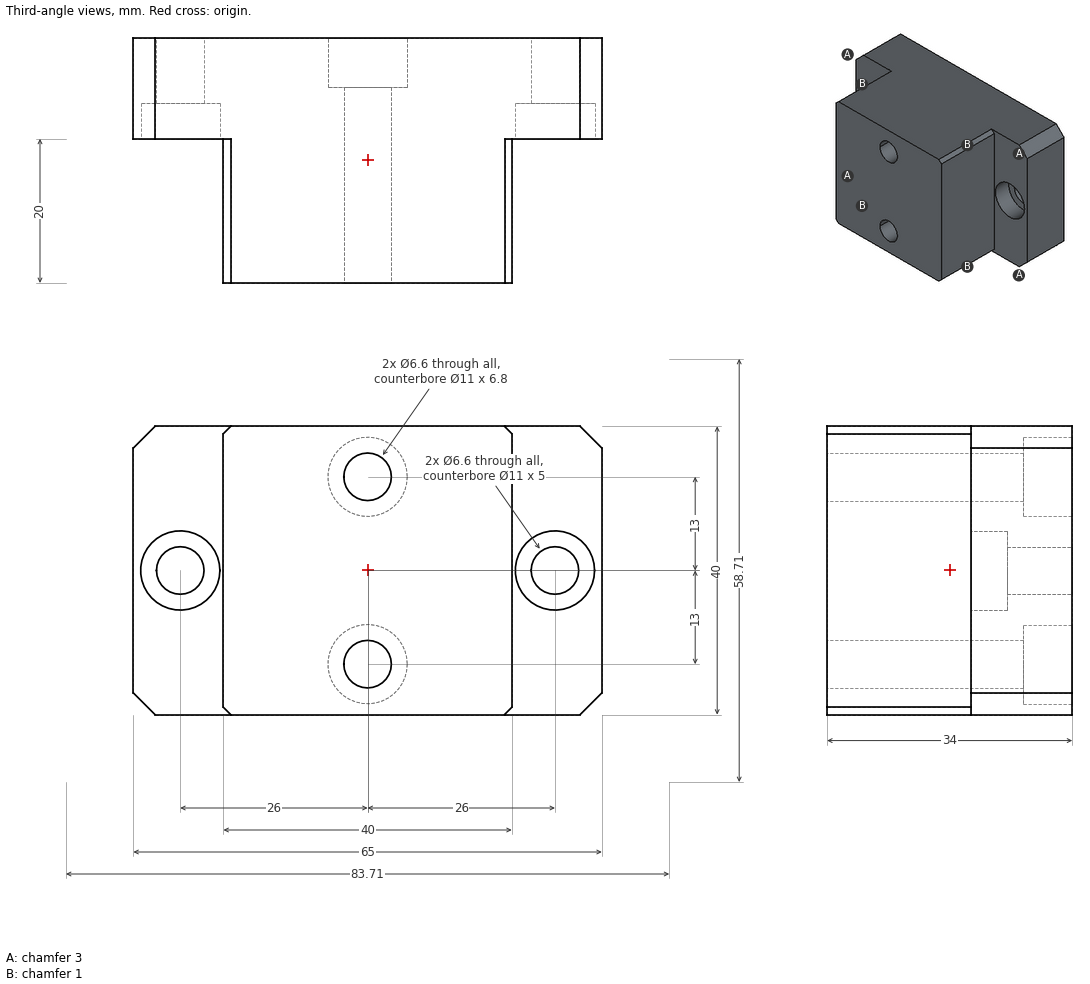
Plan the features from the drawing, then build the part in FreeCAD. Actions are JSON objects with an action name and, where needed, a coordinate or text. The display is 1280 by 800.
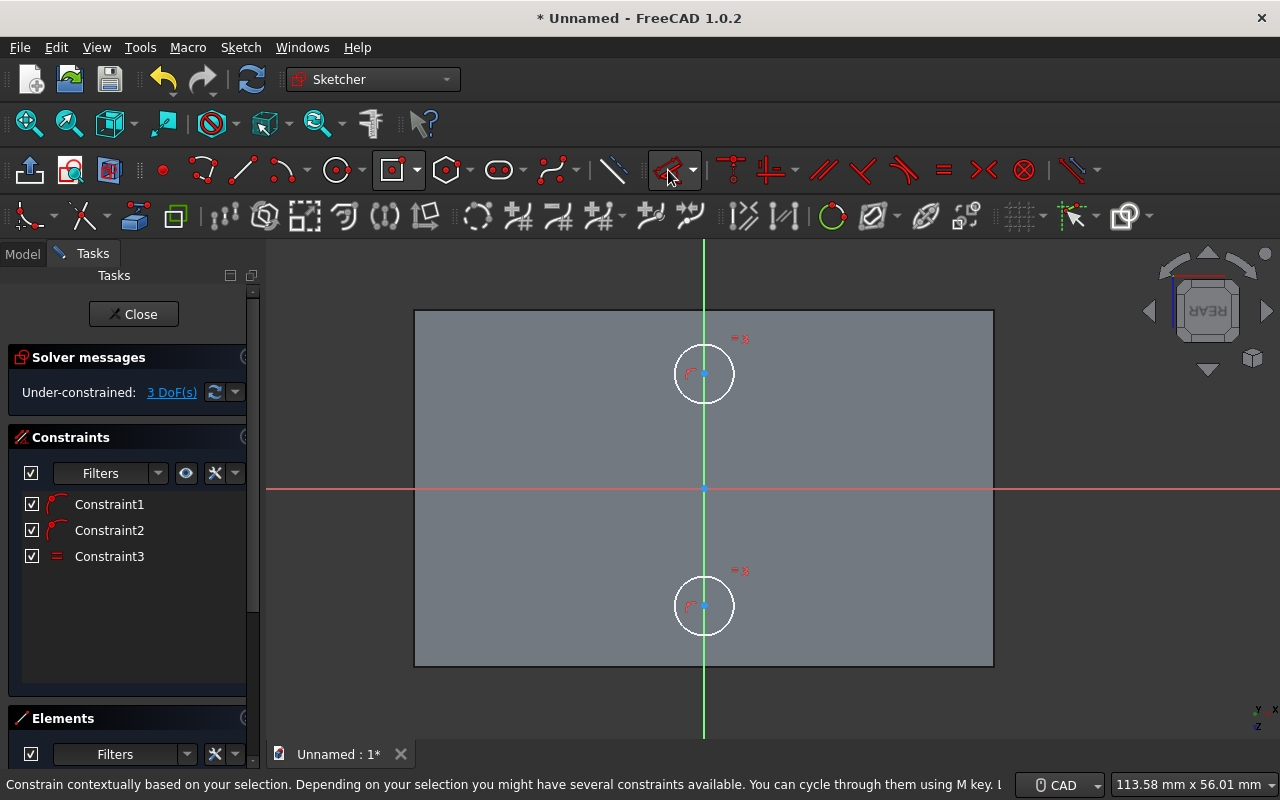
{"action": "left_click", "coordinate": [725, 585]}
{"action": "left_click", "coordinate": [747, 562]}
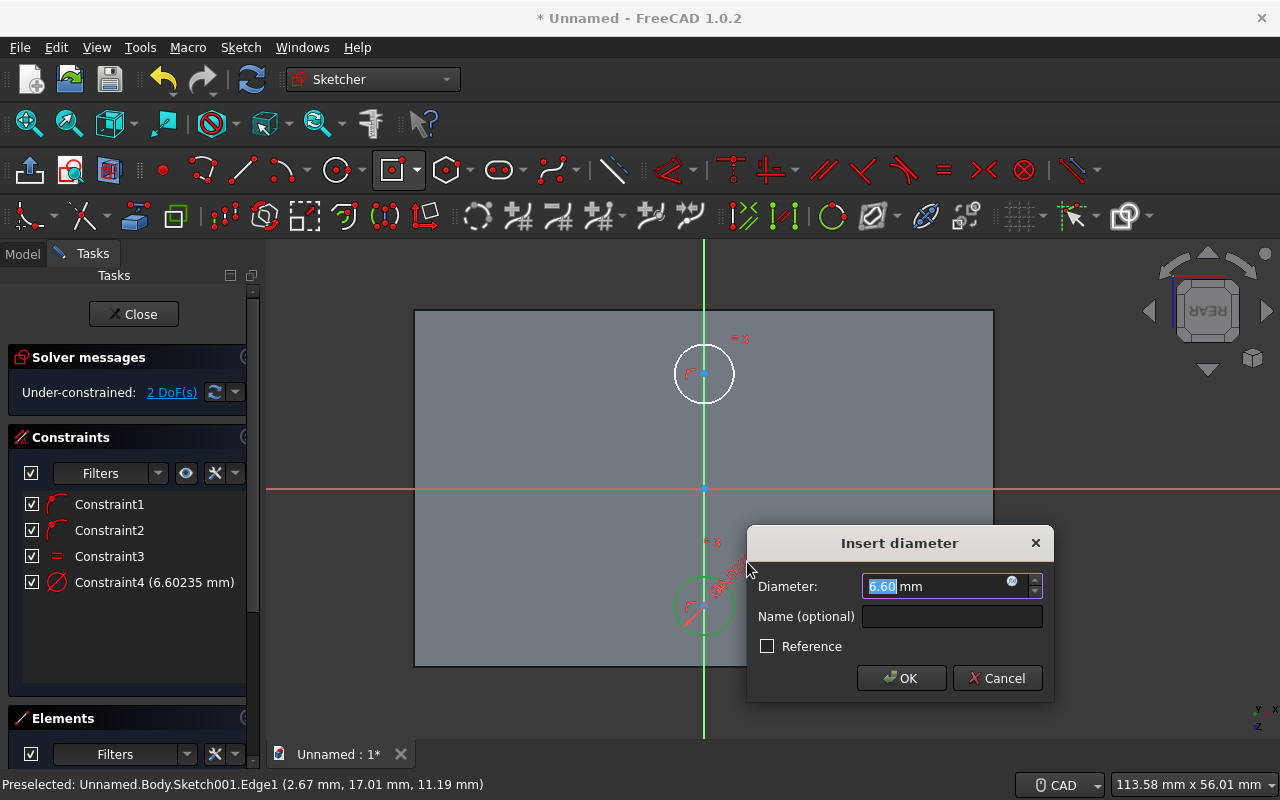
{"action": "type", "text": "6.6"}
{"action": "key", "text": "Return"}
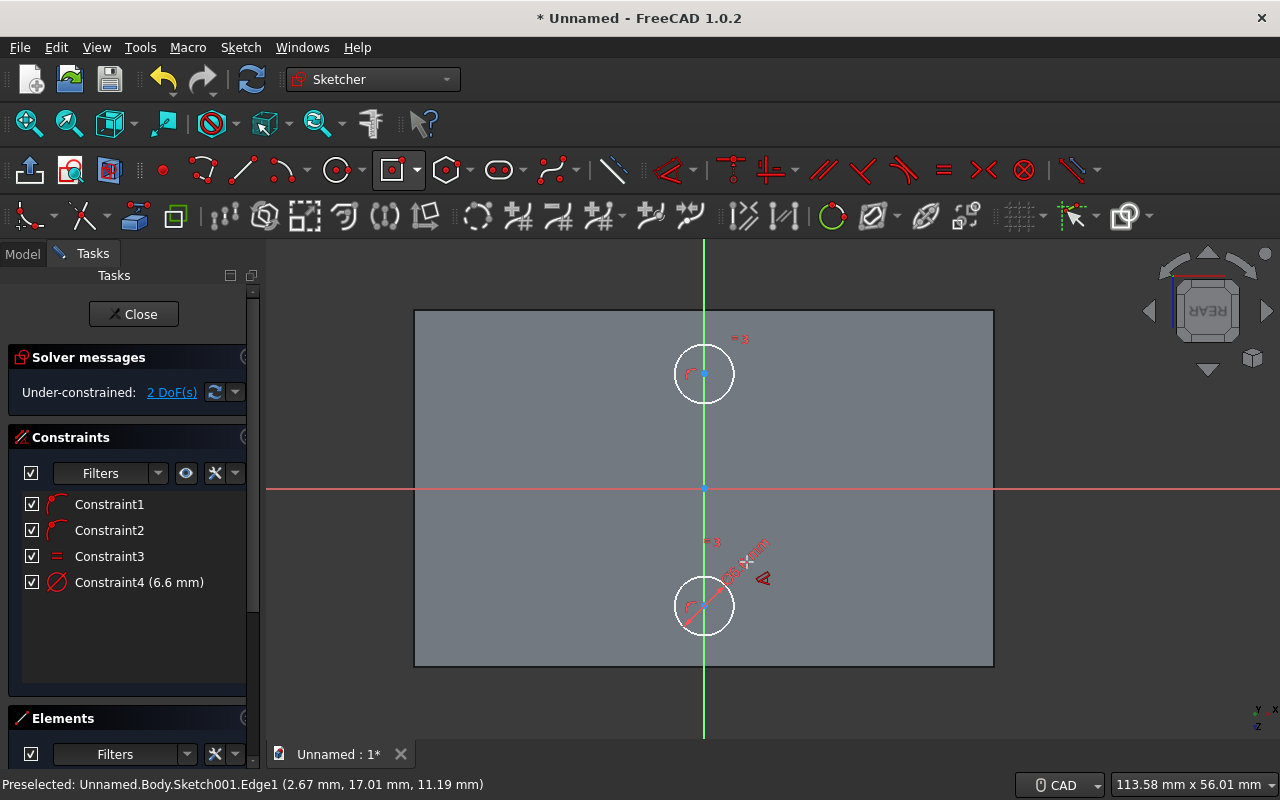
{"action": "left_click", "coordinate": [704, 606]}
{"action": "left_click", "coordinate": [738, 520]}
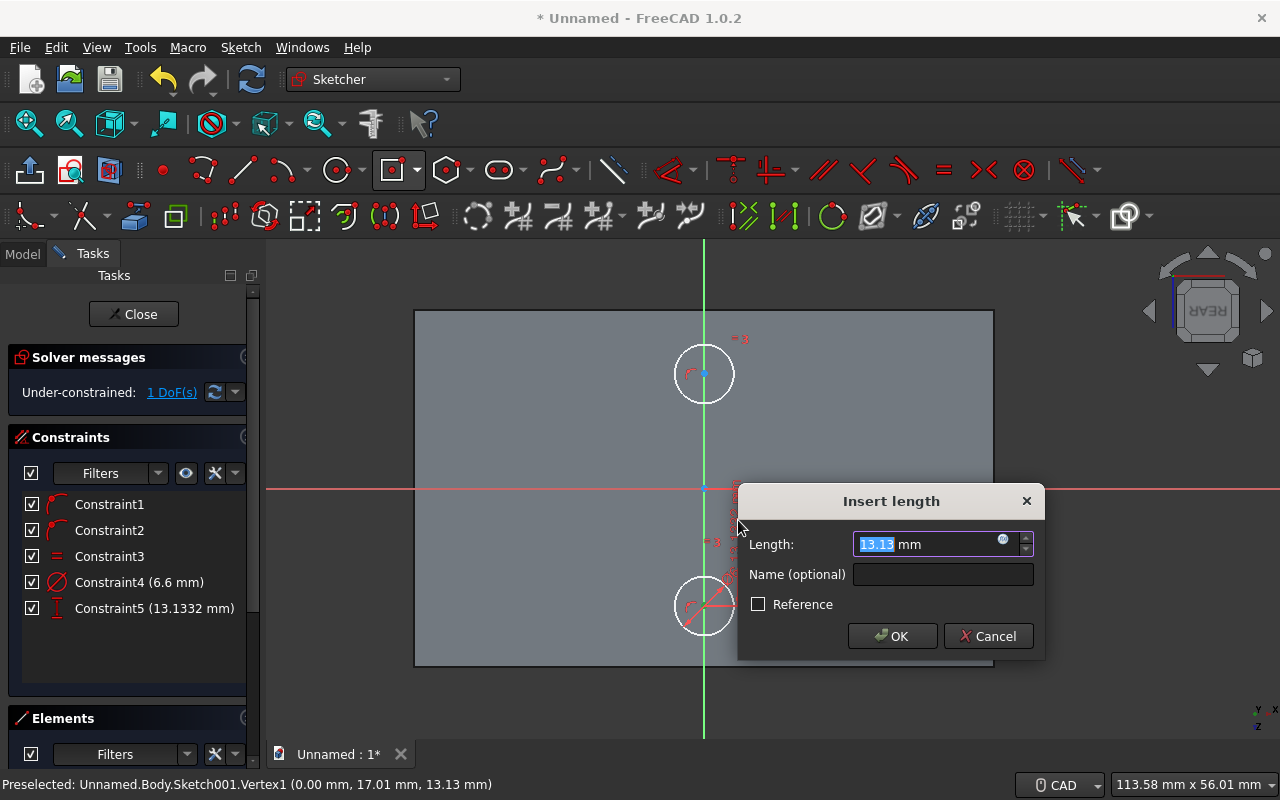
{"action": "type", "text": "13"}
{"action": "key", "text": "Return"}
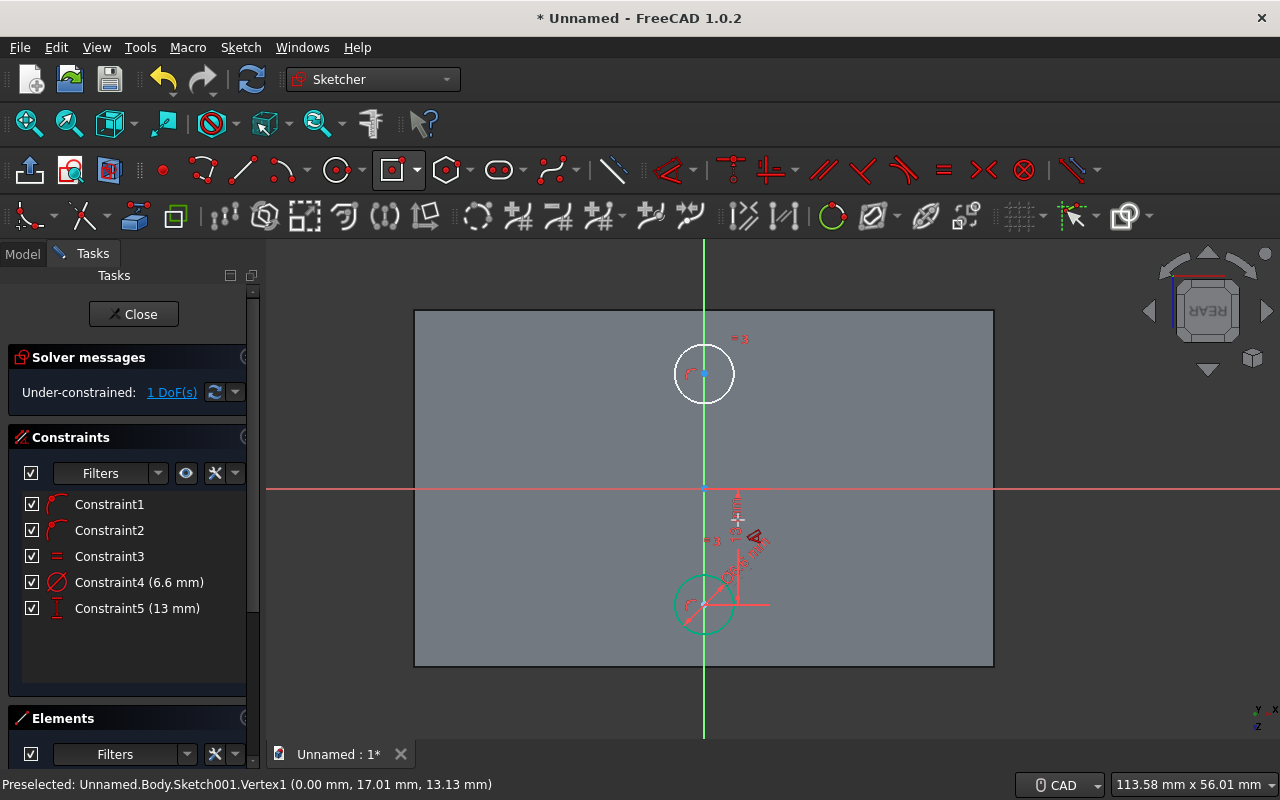
{"action": "left_click", "coordinate": [704, 374]}
{"action": "left_click", "coordinate": [738, 431]}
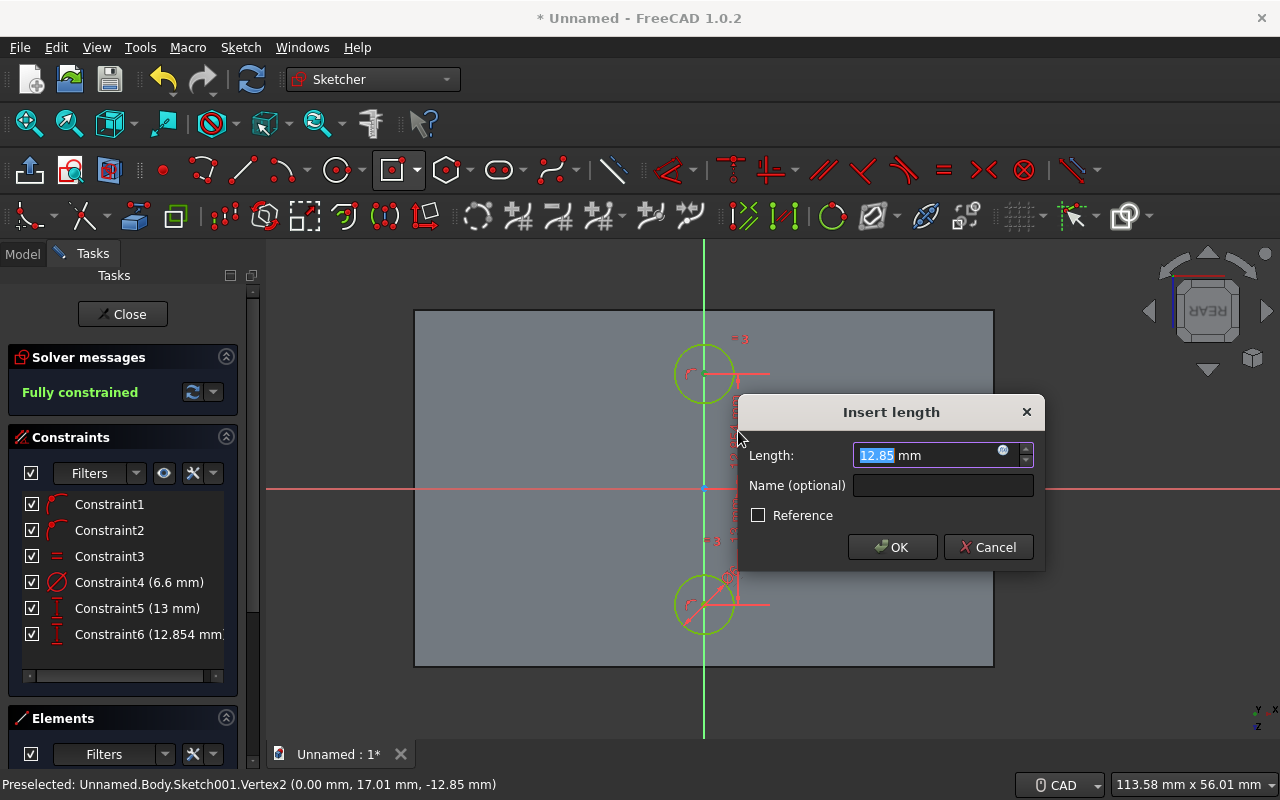
{"action": "type", "text": "13"}
{"action": "key", "text": "Return"}
{"action": "key", "text": "Escape"}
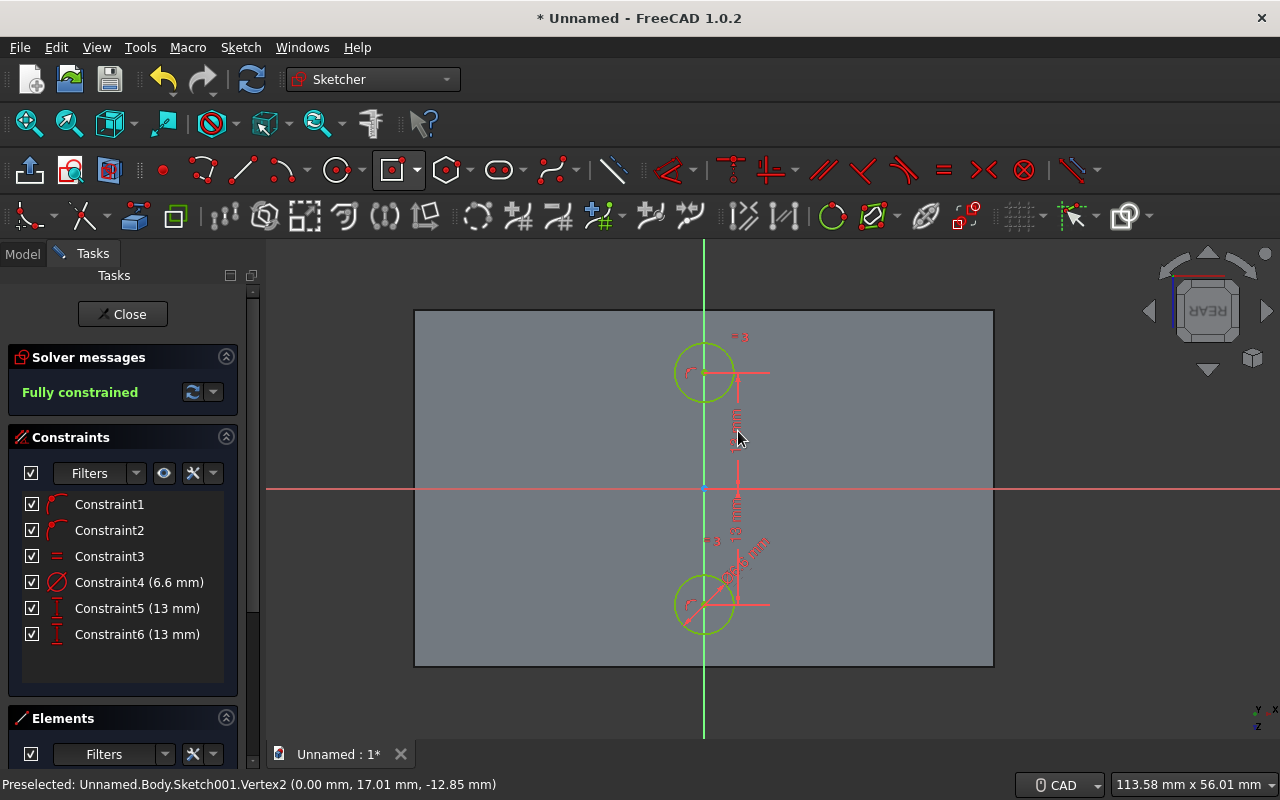
{"action": "left_click", "coordinate": [123, 314]}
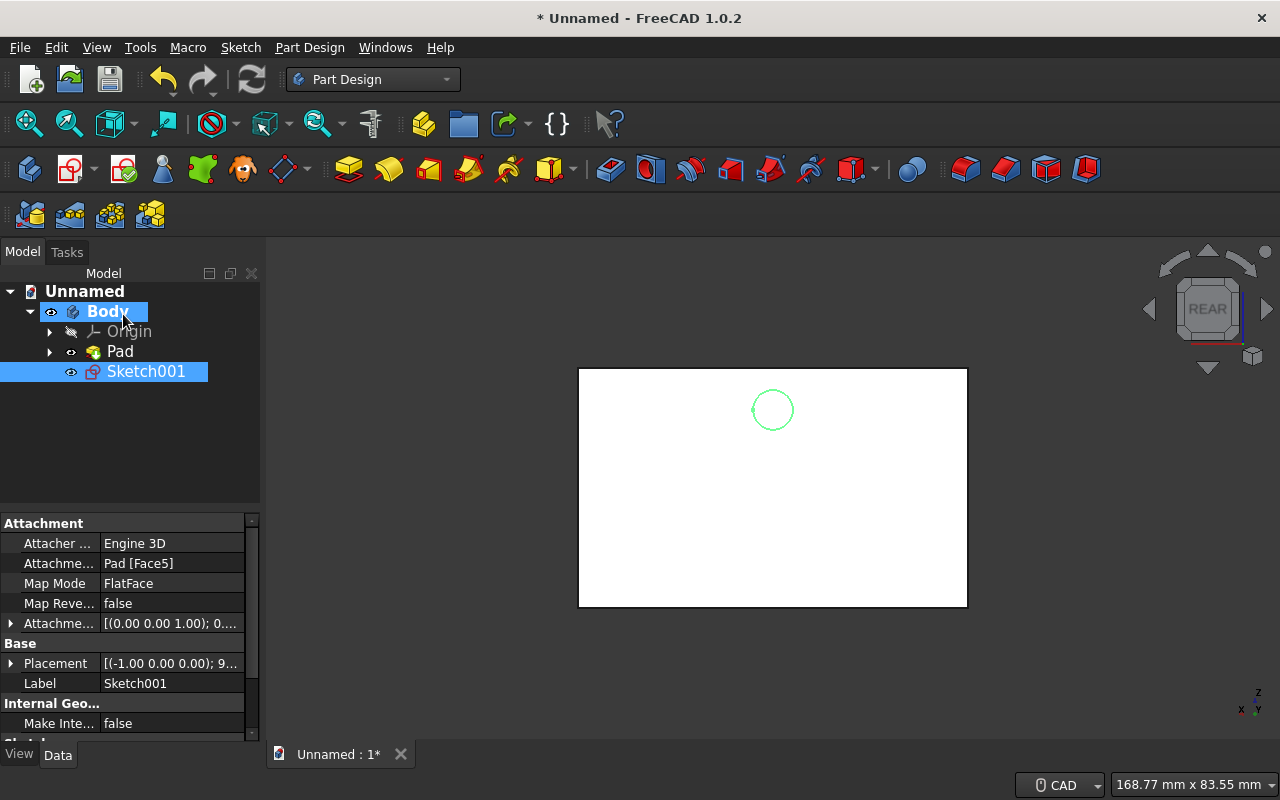
{"action": "left_click", "coordinate": [652, 170]}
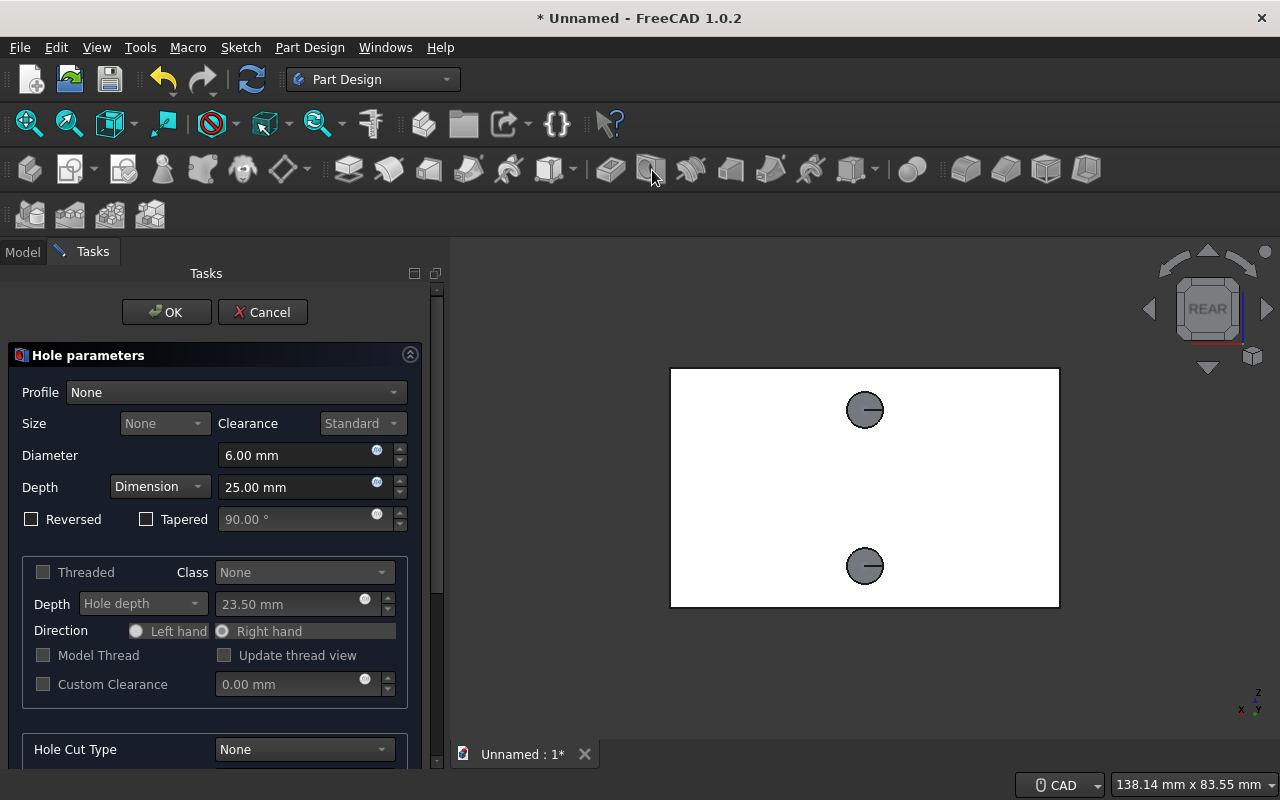
{"action": "triple_click", "coordinate": [305, 455]}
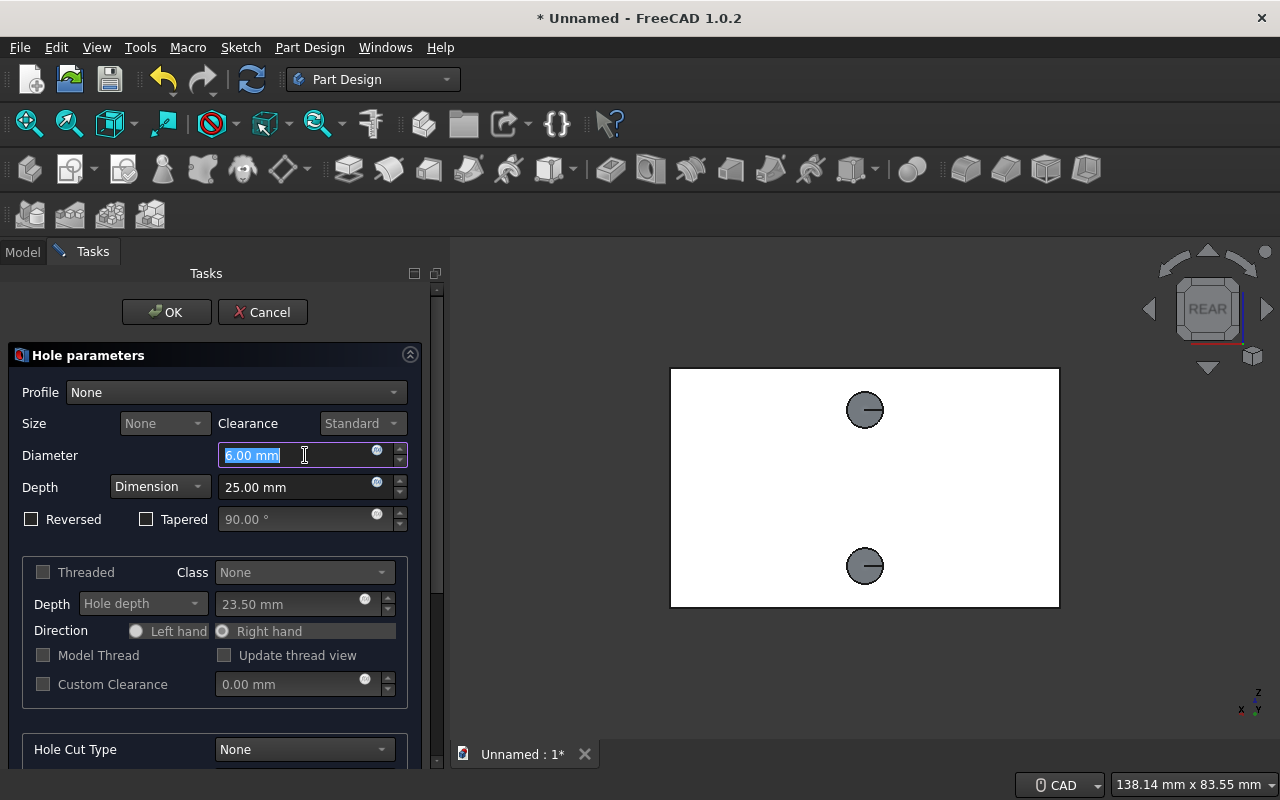
{"action": "type", "text": "6.6"}
{"action": "key", "text": "Tab"}